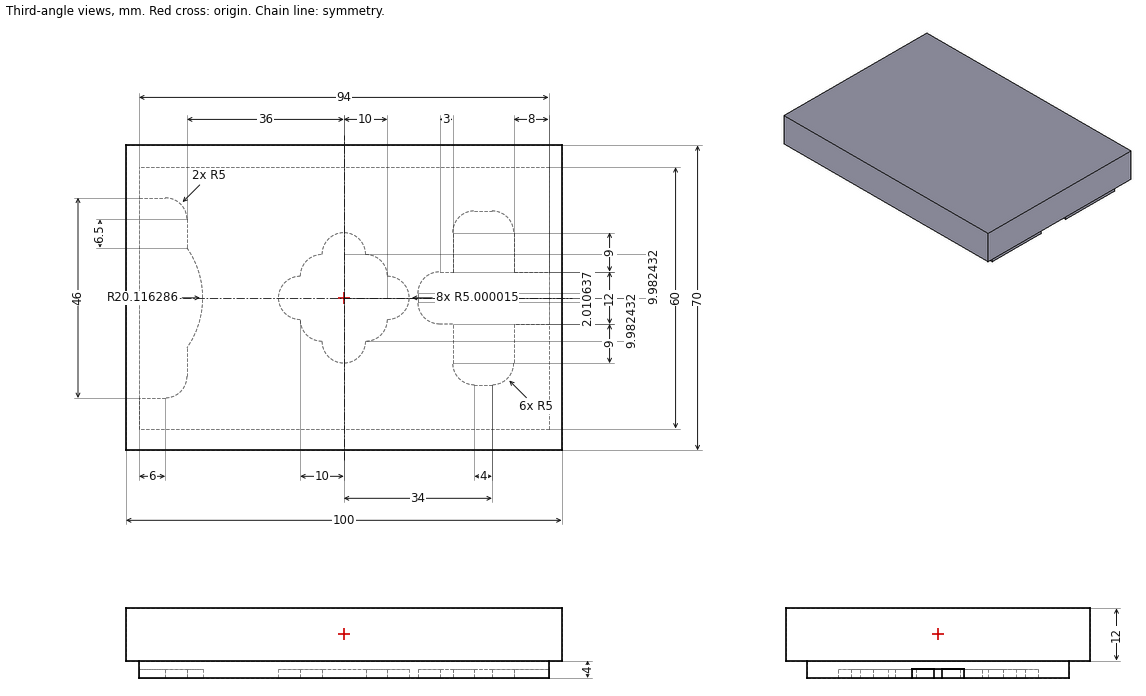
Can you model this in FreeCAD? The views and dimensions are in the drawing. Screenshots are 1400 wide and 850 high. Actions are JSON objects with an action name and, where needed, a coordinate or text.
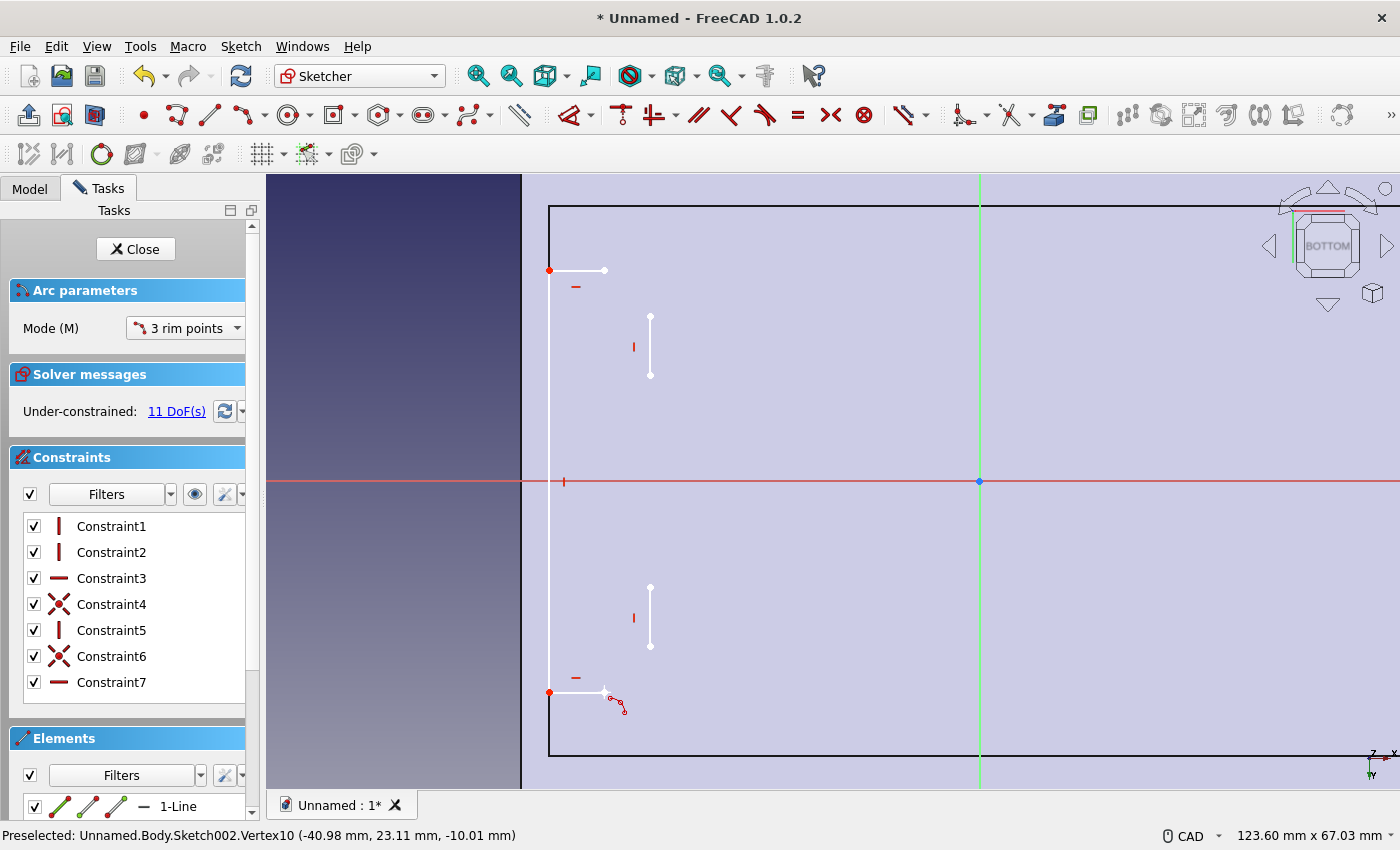
{"action": "left_click", "coordinate": [650, 588]}
{"action": "left_click", "coordinate": [650, 376]}
{"action": "left_click", "coordinate": [681, 503]}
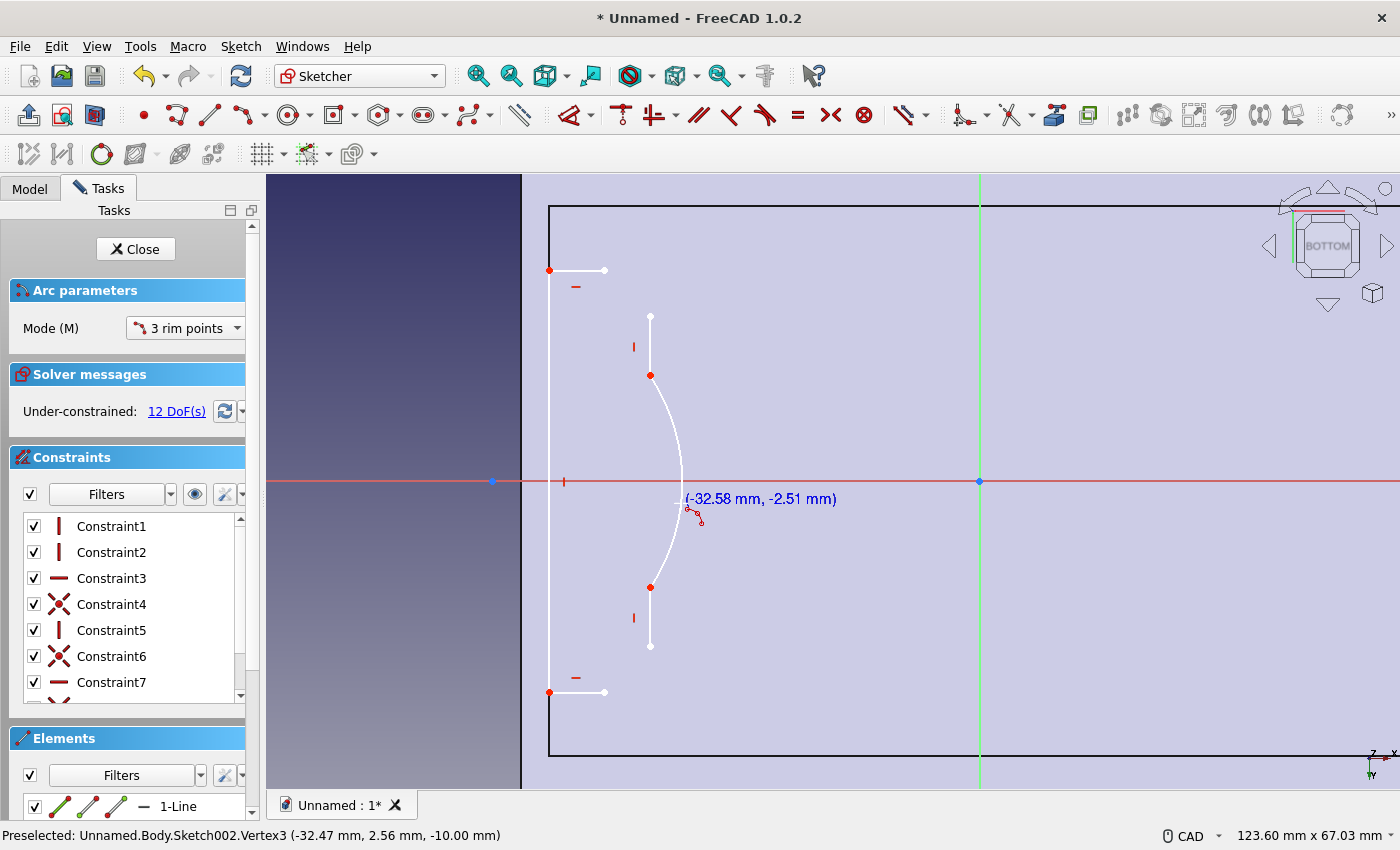
{"action": "left_click", "coordinate": [650, 317]}
{"action": "left_click", "coordinate": [604, 271]}
{"action": "left_click", "coordinate": [636, 283]}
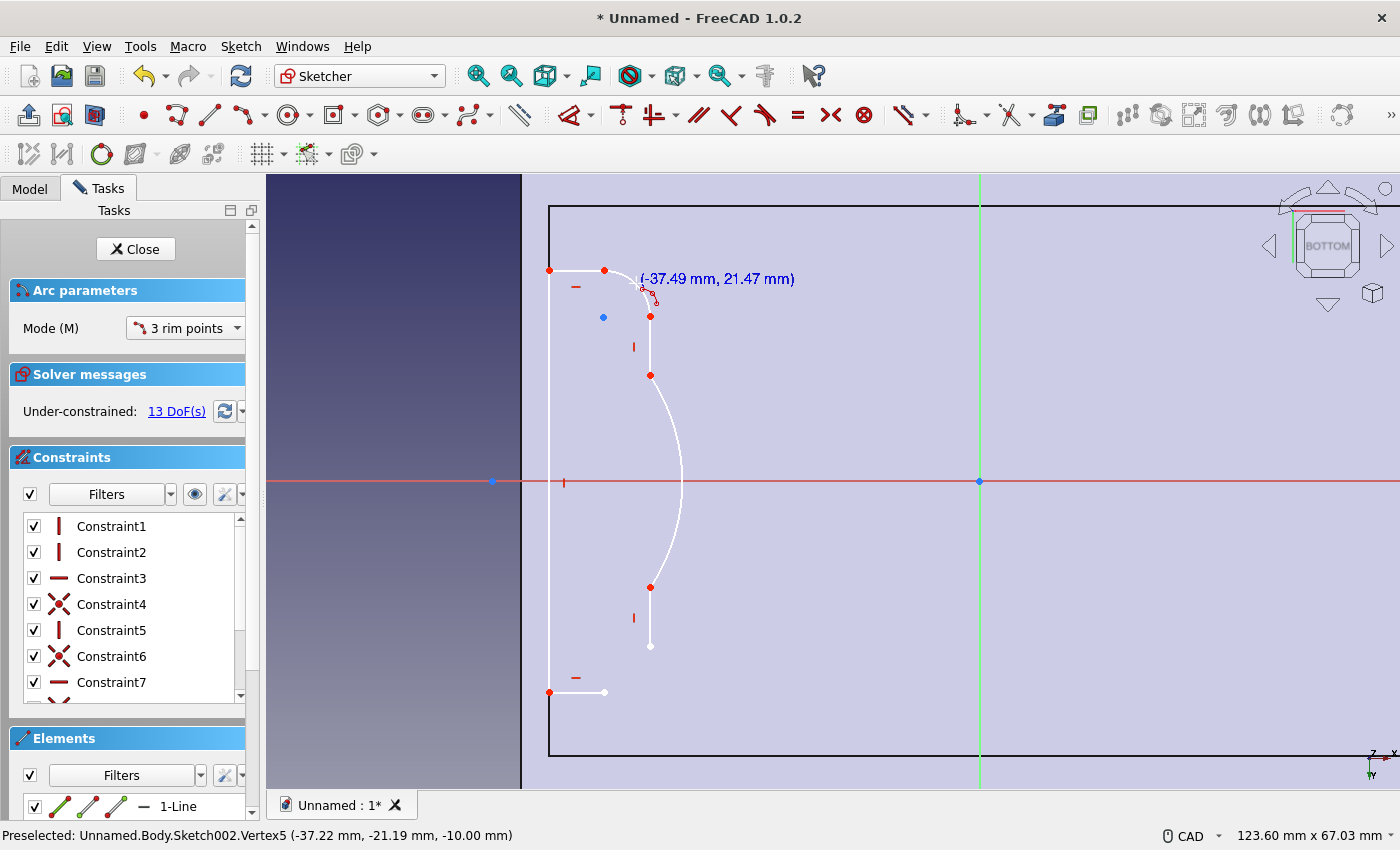
{"action": "left_click", "coordinate": [604, 693]}
{"action": "left_click", "coordinate": [650, 647]}
{"action": "left_click", "coordinate": [636, 679]}
{"action": "key", "text": "Escape"}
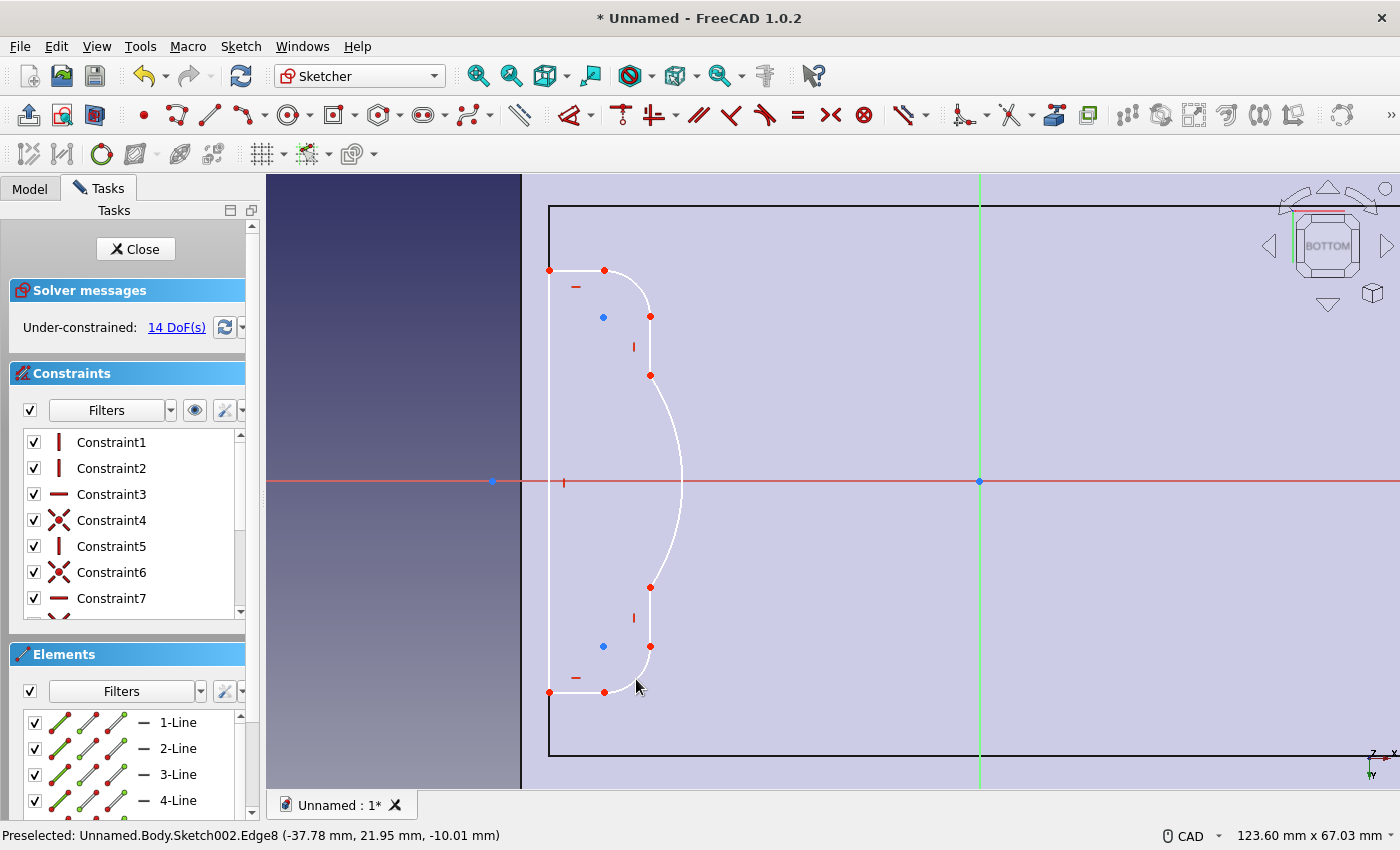
{"action": "left_click", "coordinate": [650, 629]}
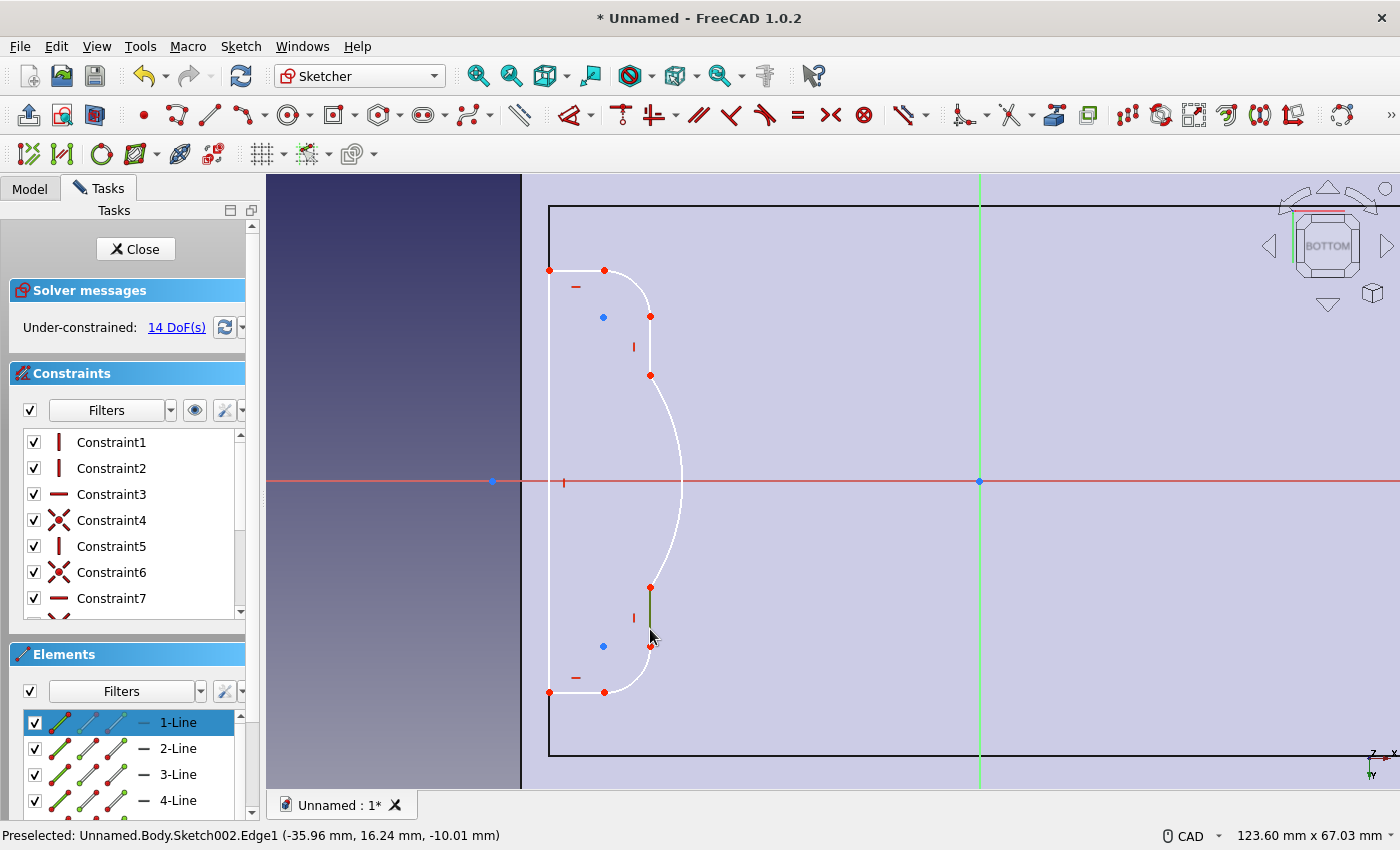
{"action": "left_click", "coordinate": [625, 688]}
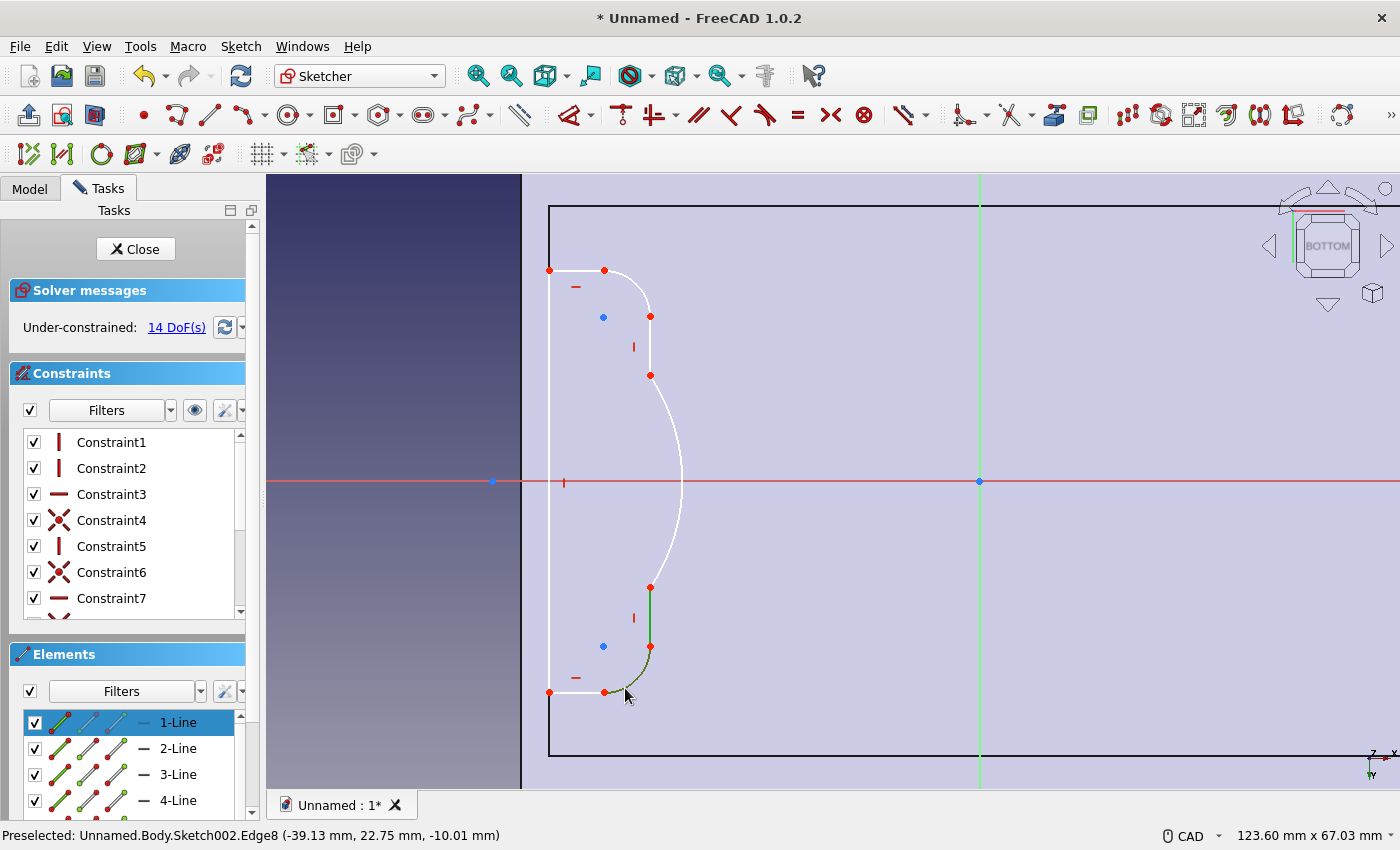
{"action": "left_click", "coordinate": [765, 116]}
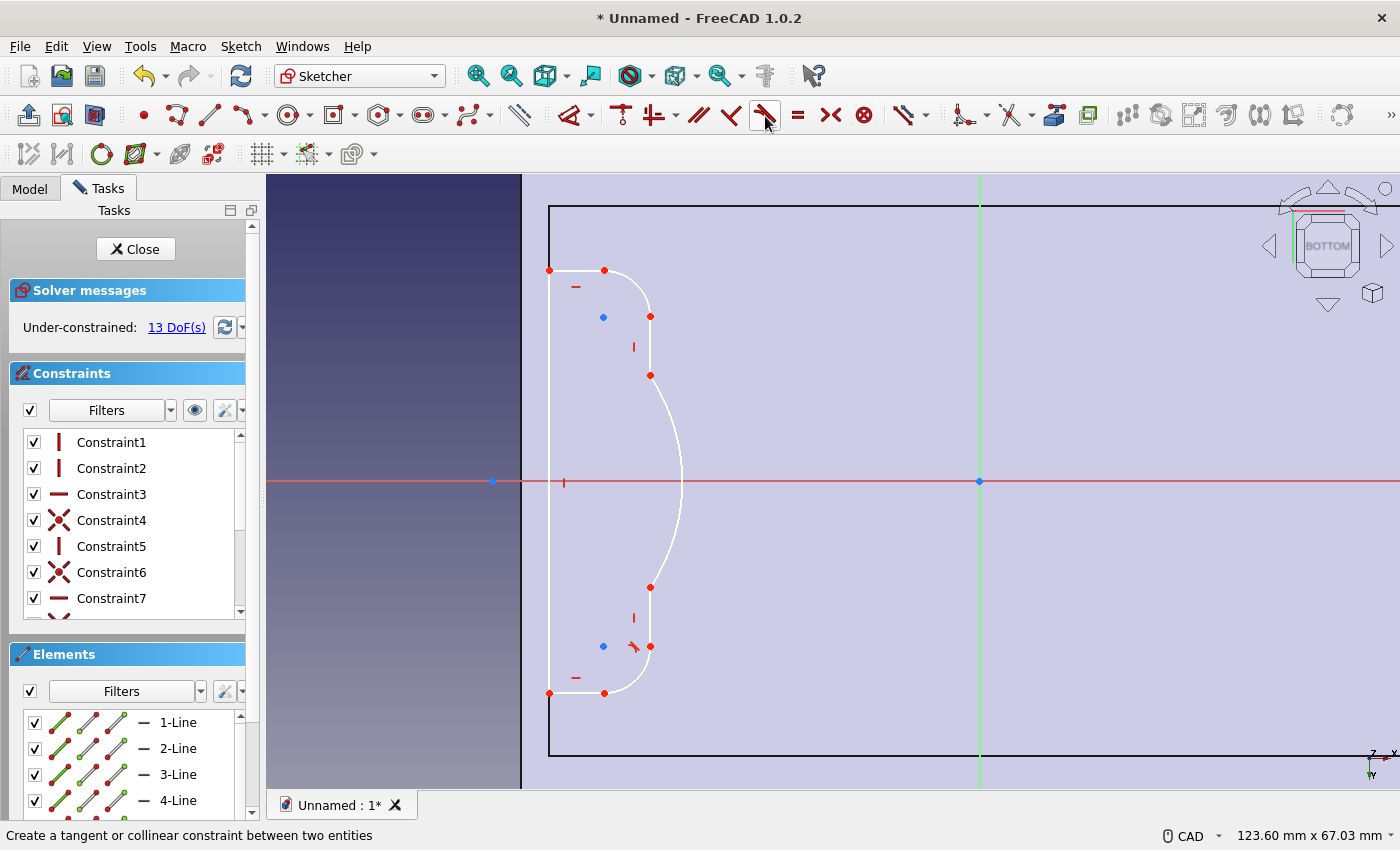
{"action": "left_click", "coordinate": [650, 358]}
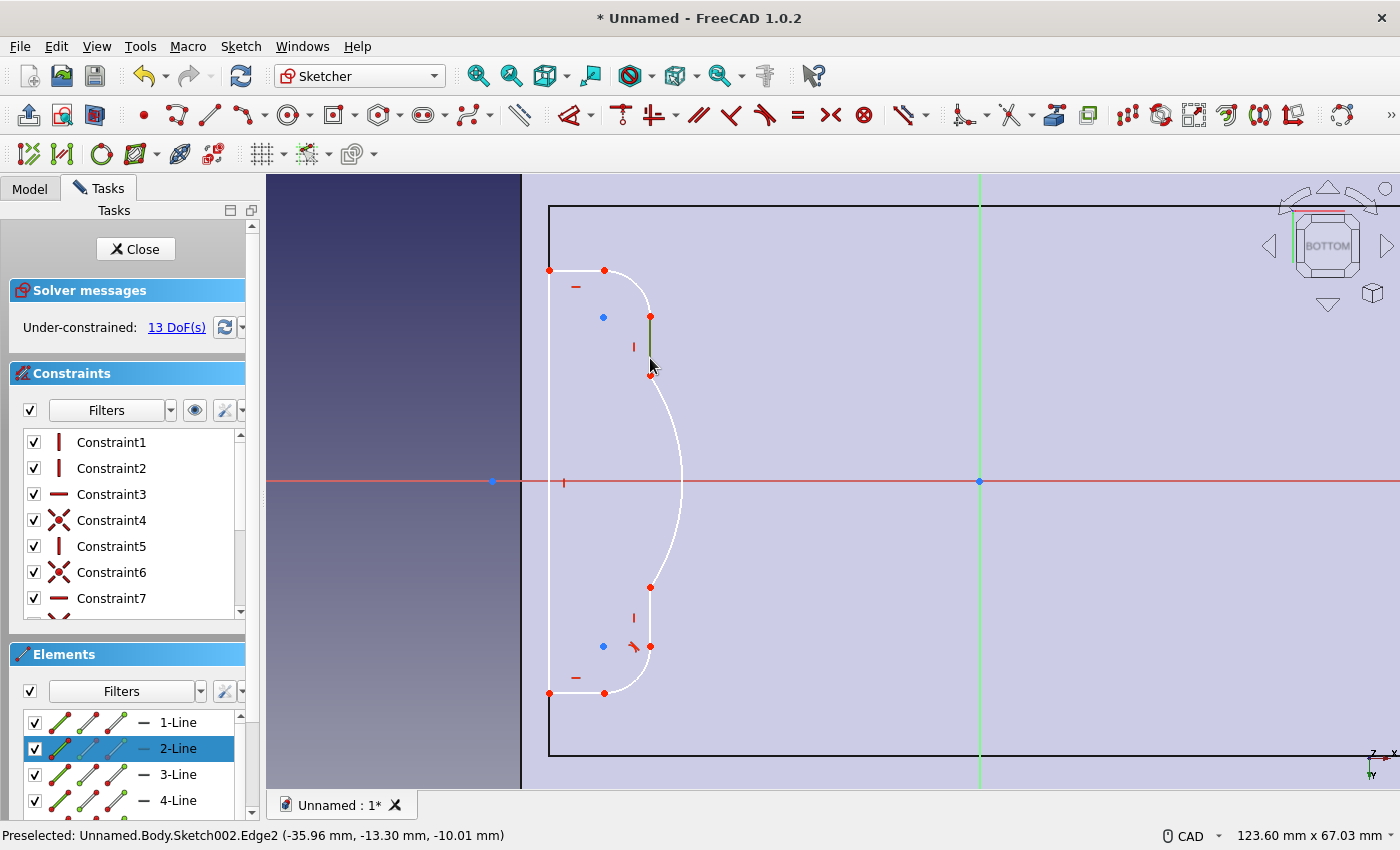
{"action": "left_click", "coordinate": [645, 296]}